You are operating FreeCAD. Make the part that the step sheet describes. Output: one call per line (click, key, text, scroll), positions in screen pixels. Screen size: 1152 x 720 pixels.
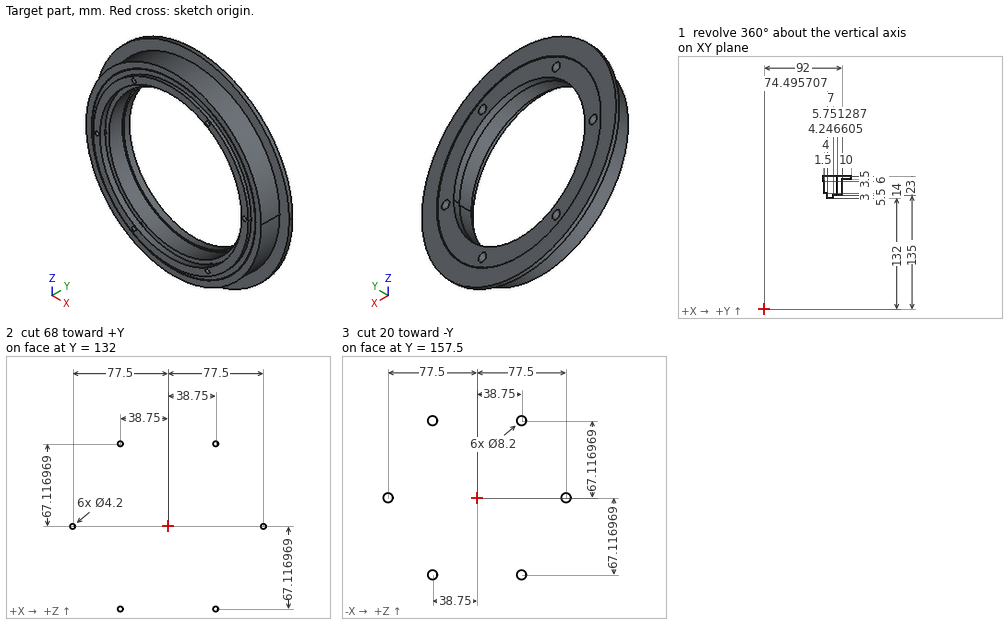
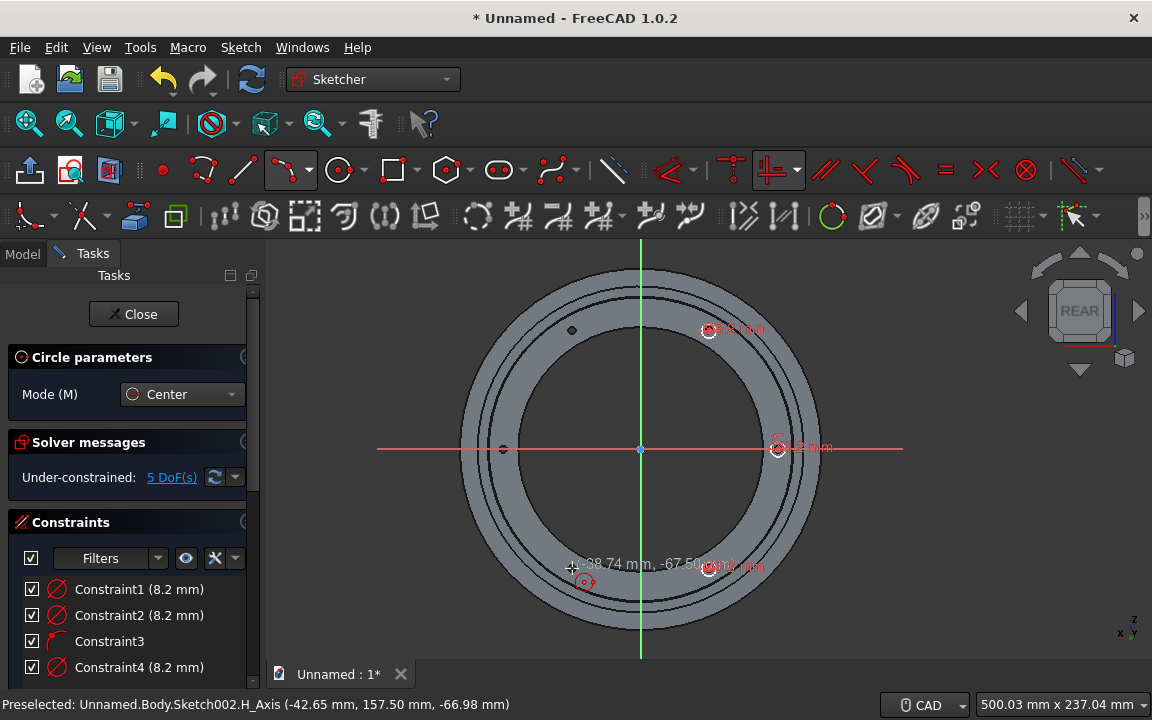
click(572, 568)
move(577, 563)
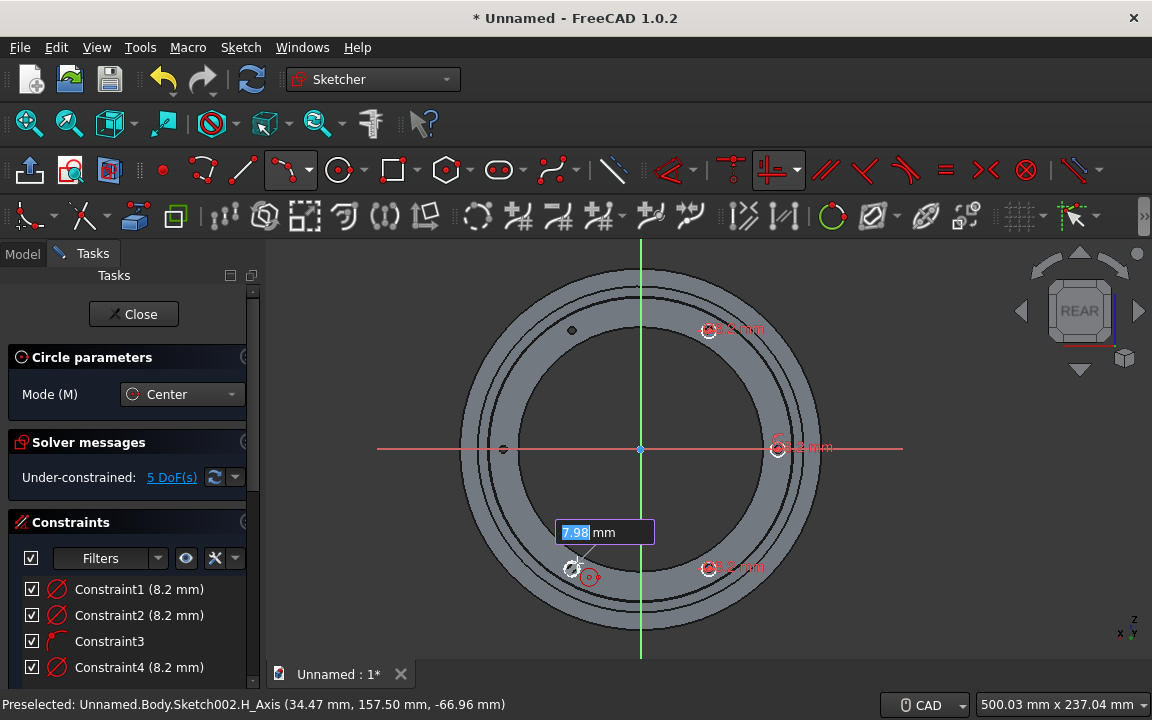
text(8.2)
key(Return)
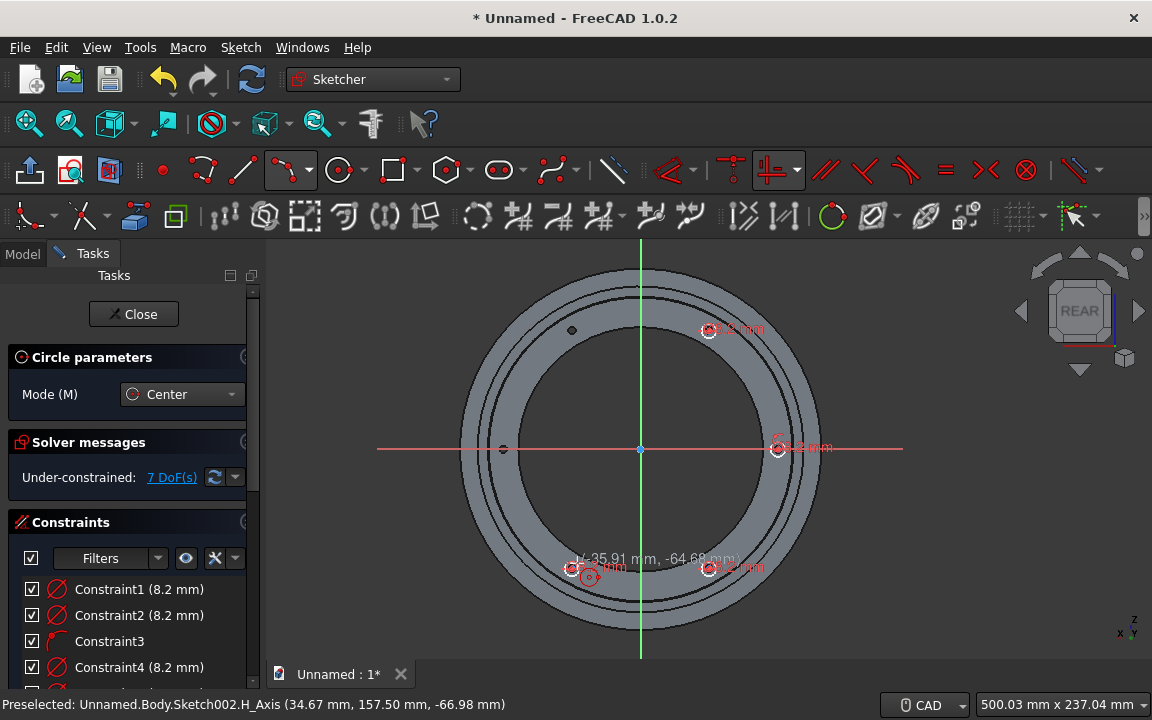
scroll(503, 449, up, 6)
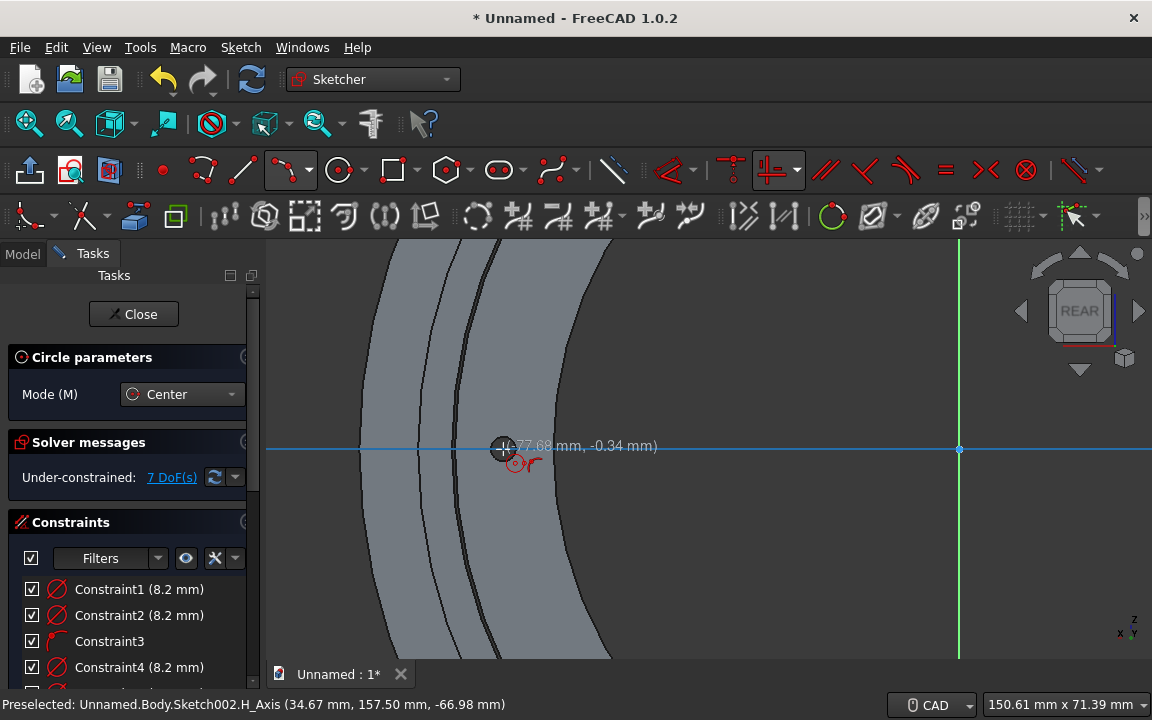
scroll(503, 449, down, 6)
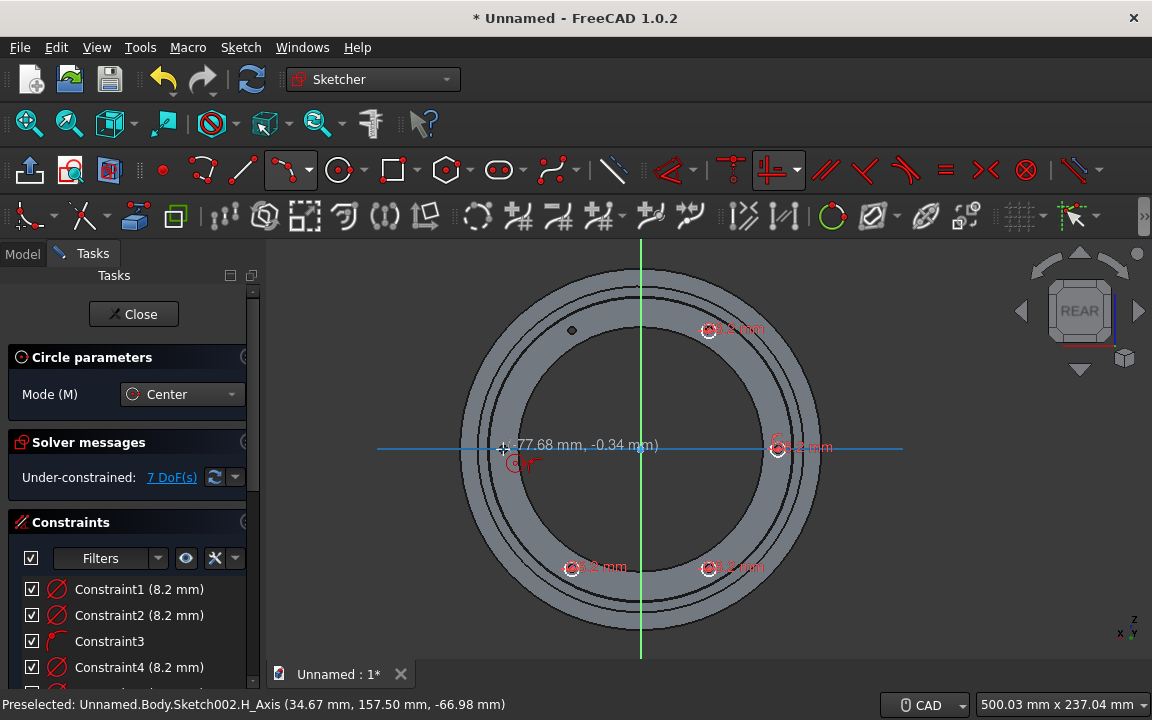
click(503, 449)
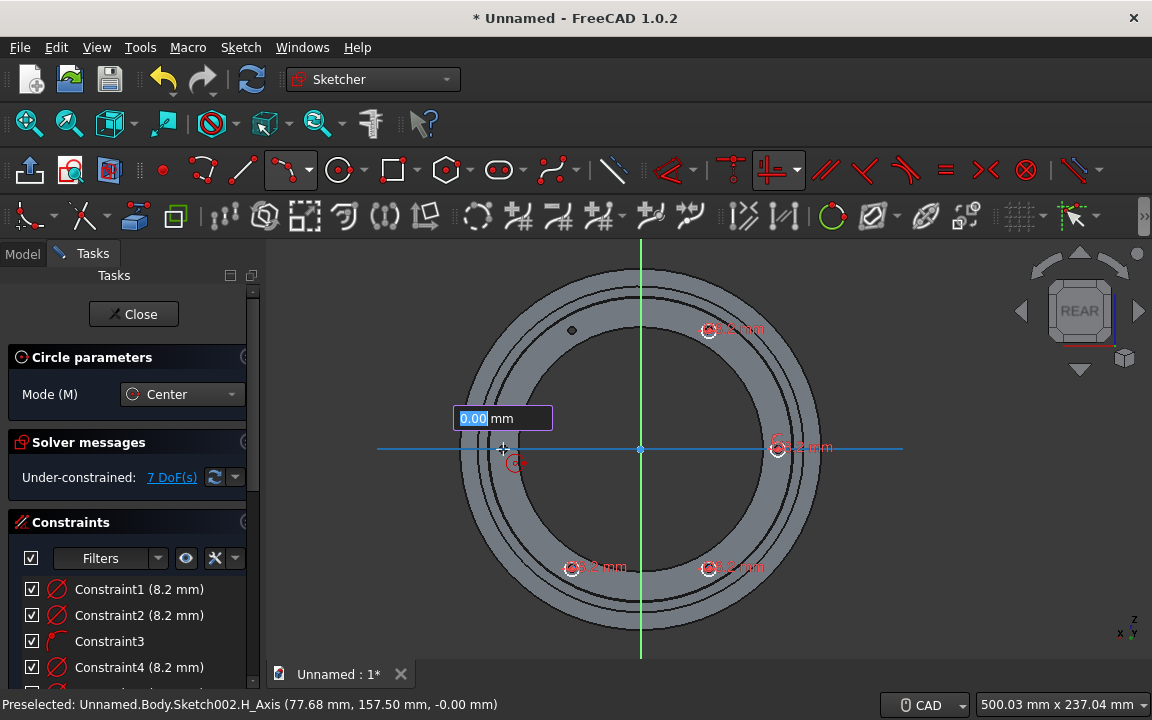
scroll(501, 456, up, 5)
move(500, 456)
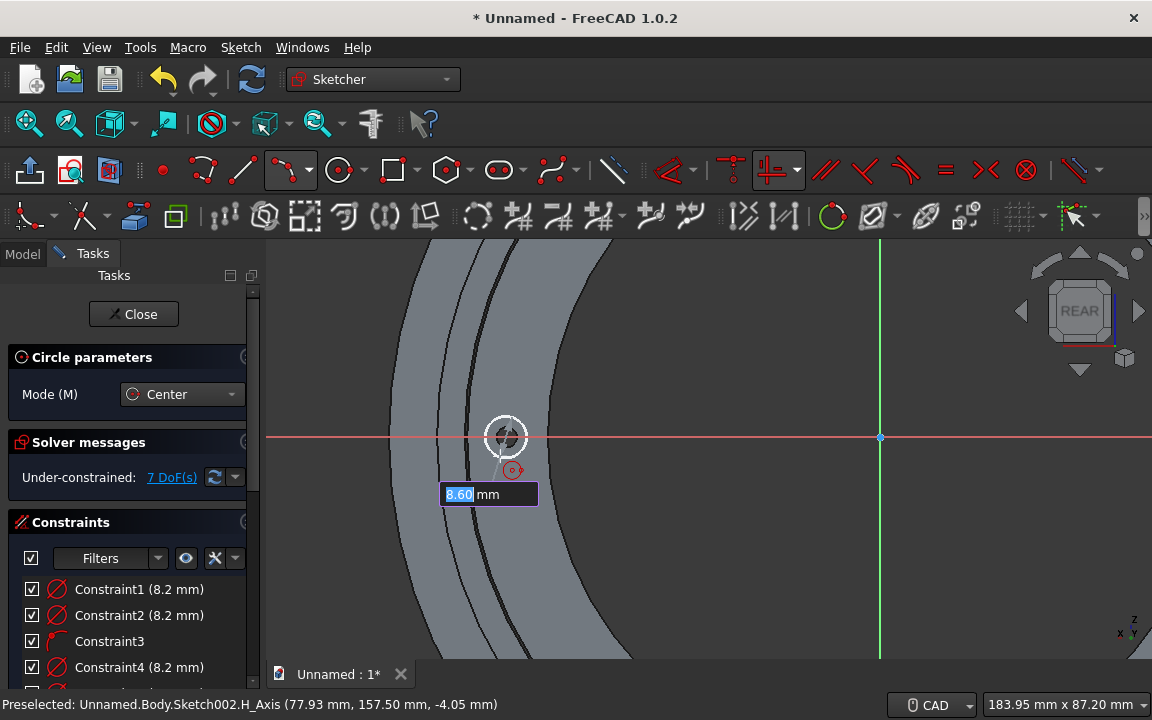
text(8.2)
key(Return)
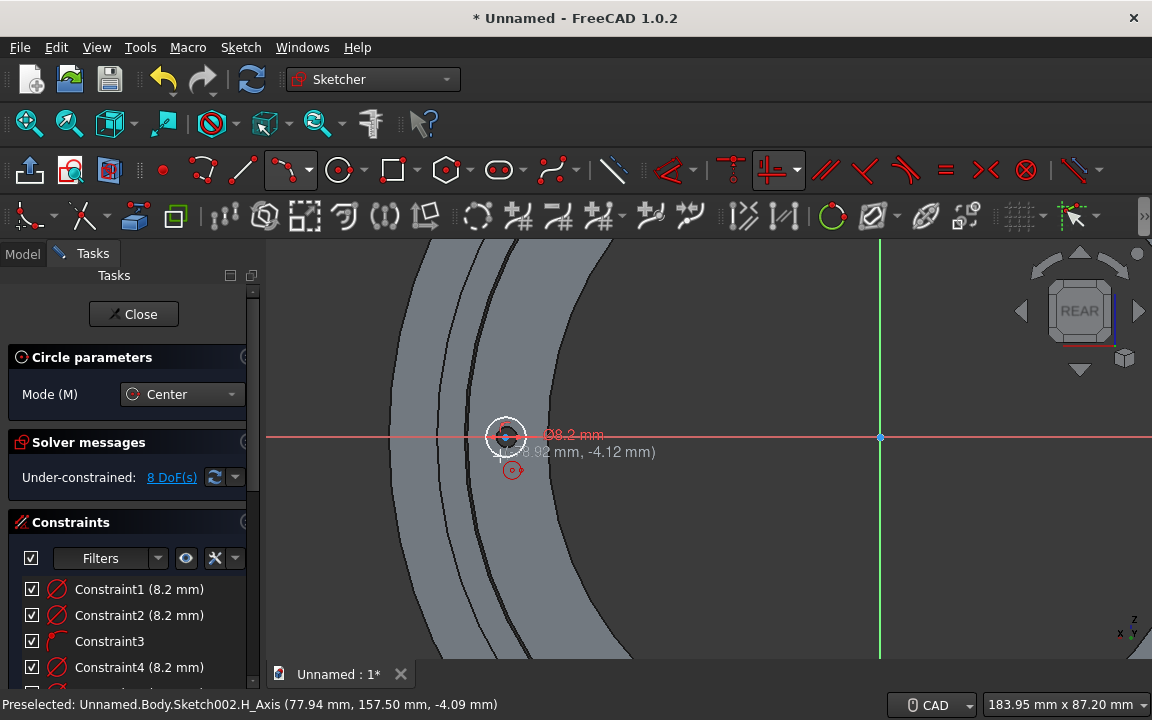
scroll(501, 456, down, 5)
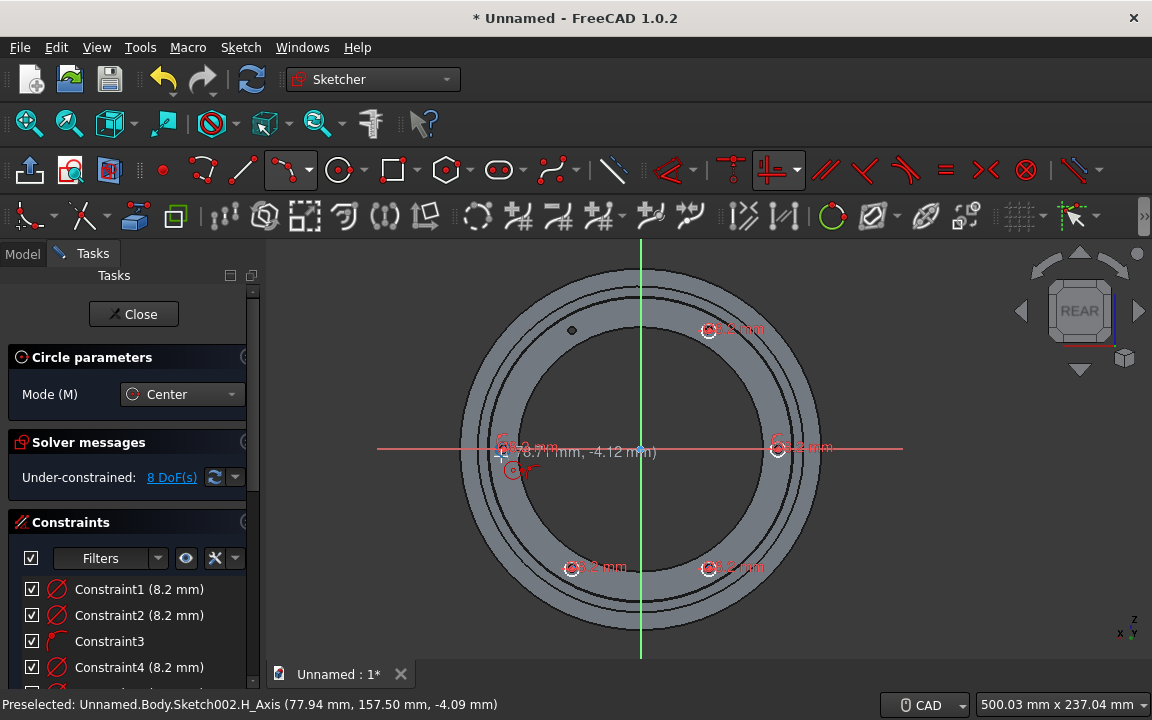
scroll(572, 330, up, 6)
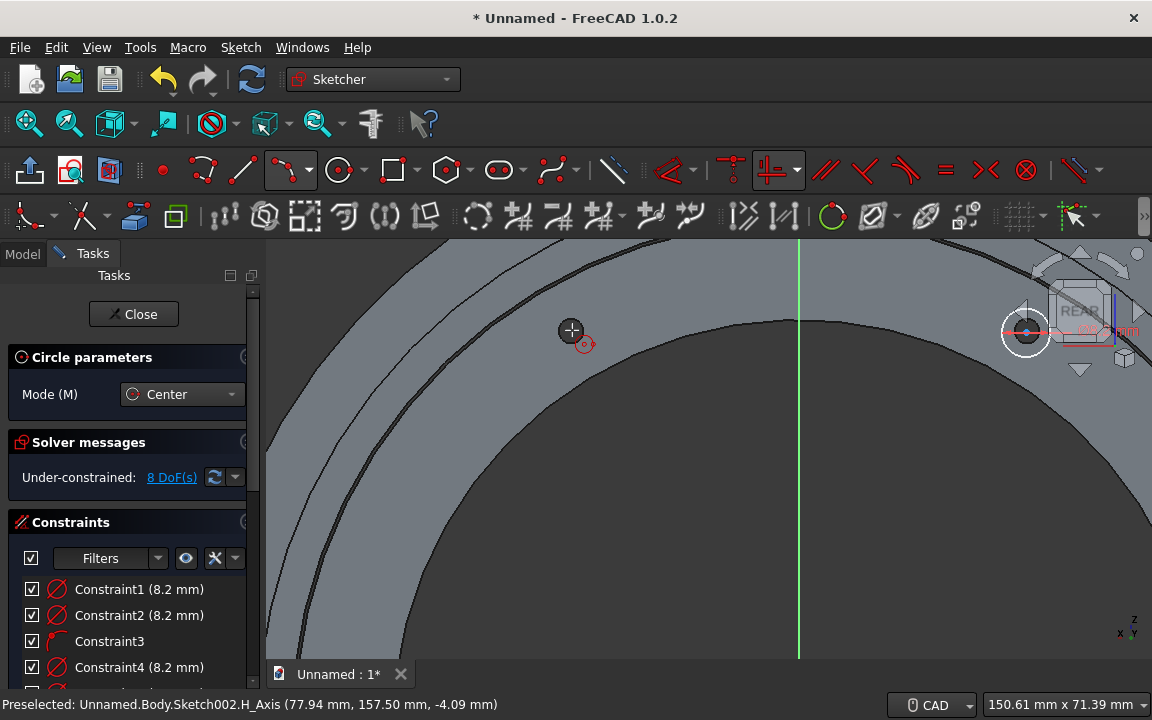
scroll(572, 330, down, 6)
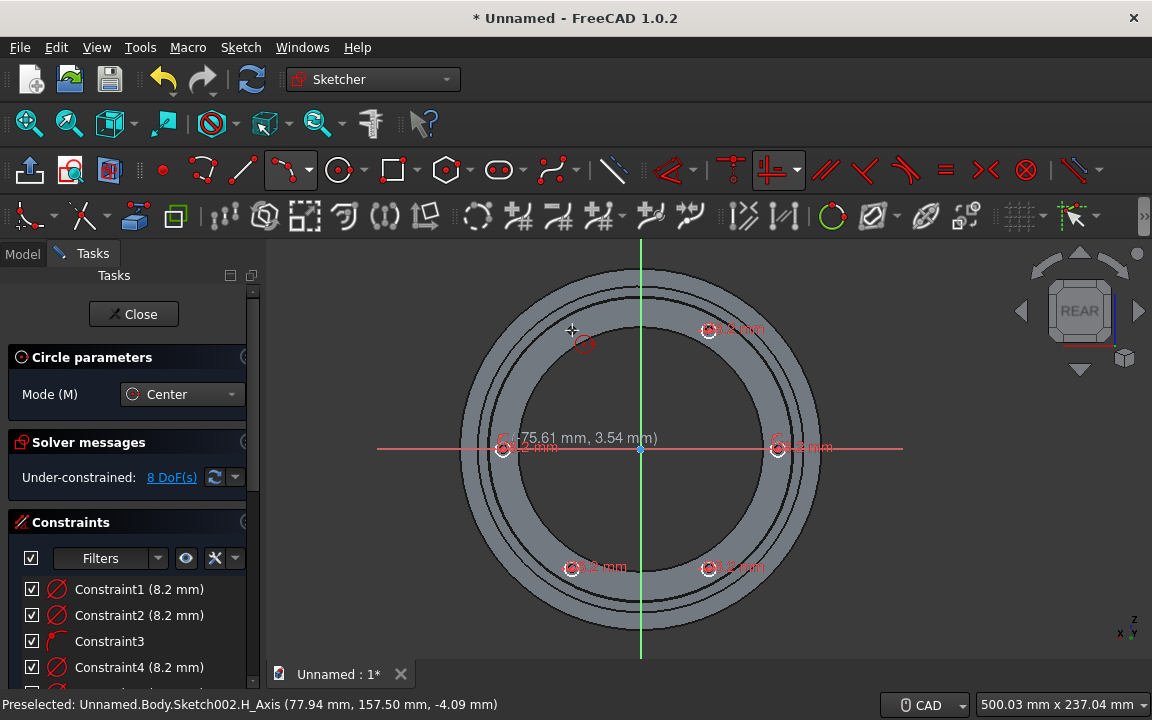
click(572, 330)
move(577, 325)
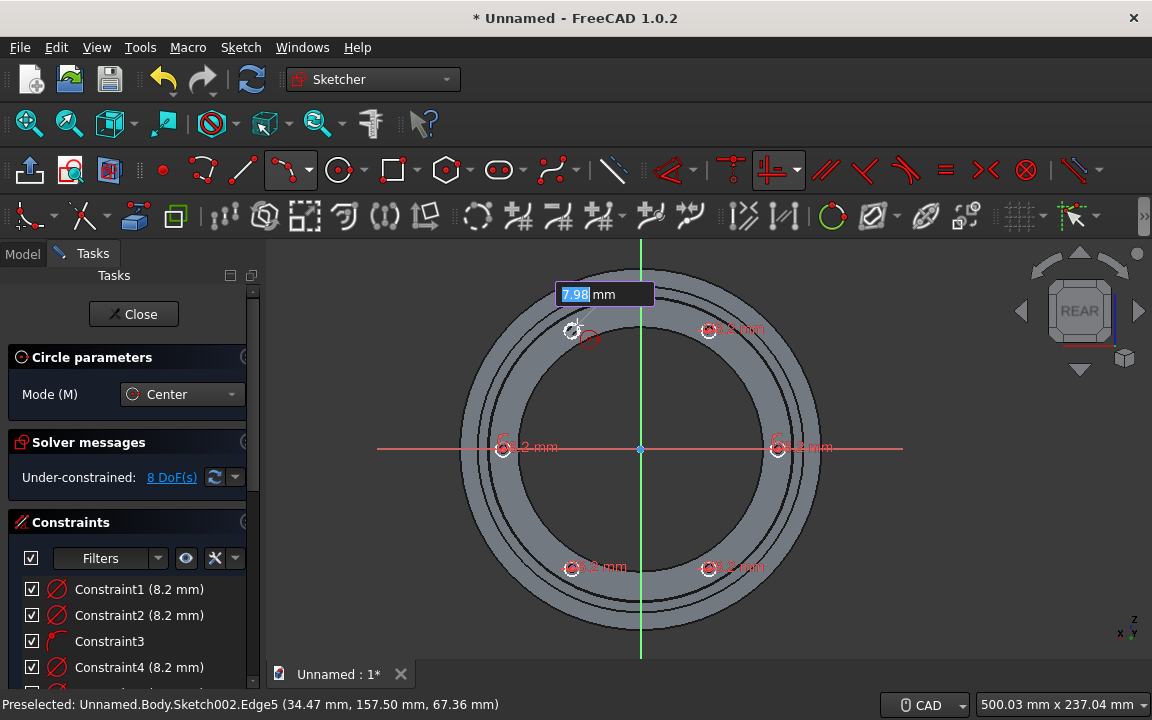
text(8.2)
key(Return)
key(Escape)